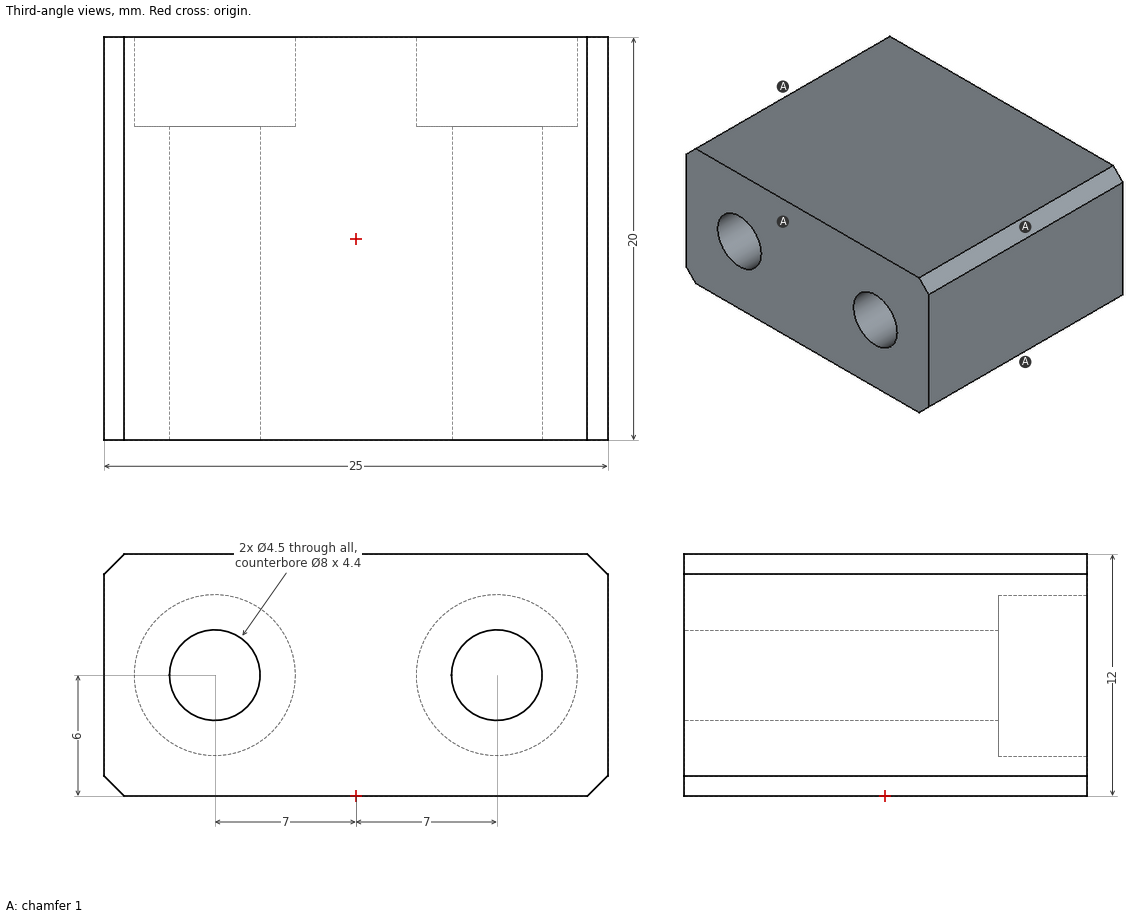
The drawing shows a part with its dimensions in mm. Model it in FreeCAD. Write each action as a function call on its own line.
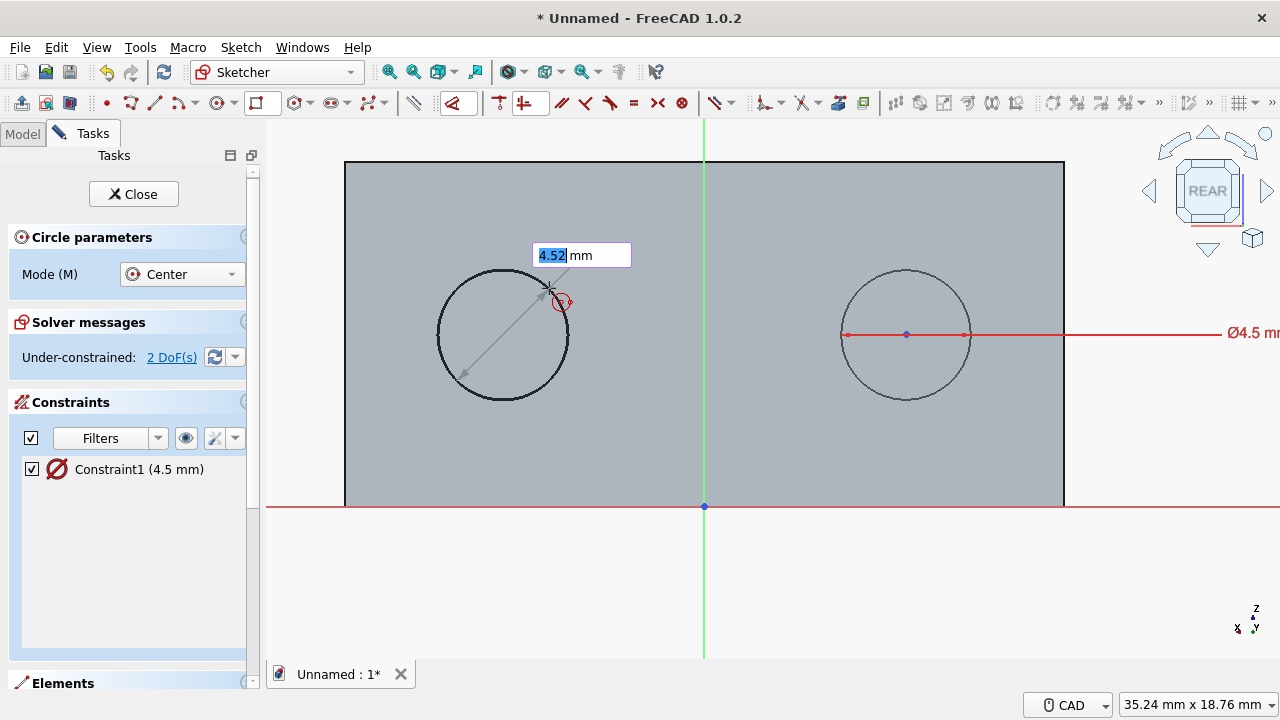
text(4.5)
key(Return)
key(Escape)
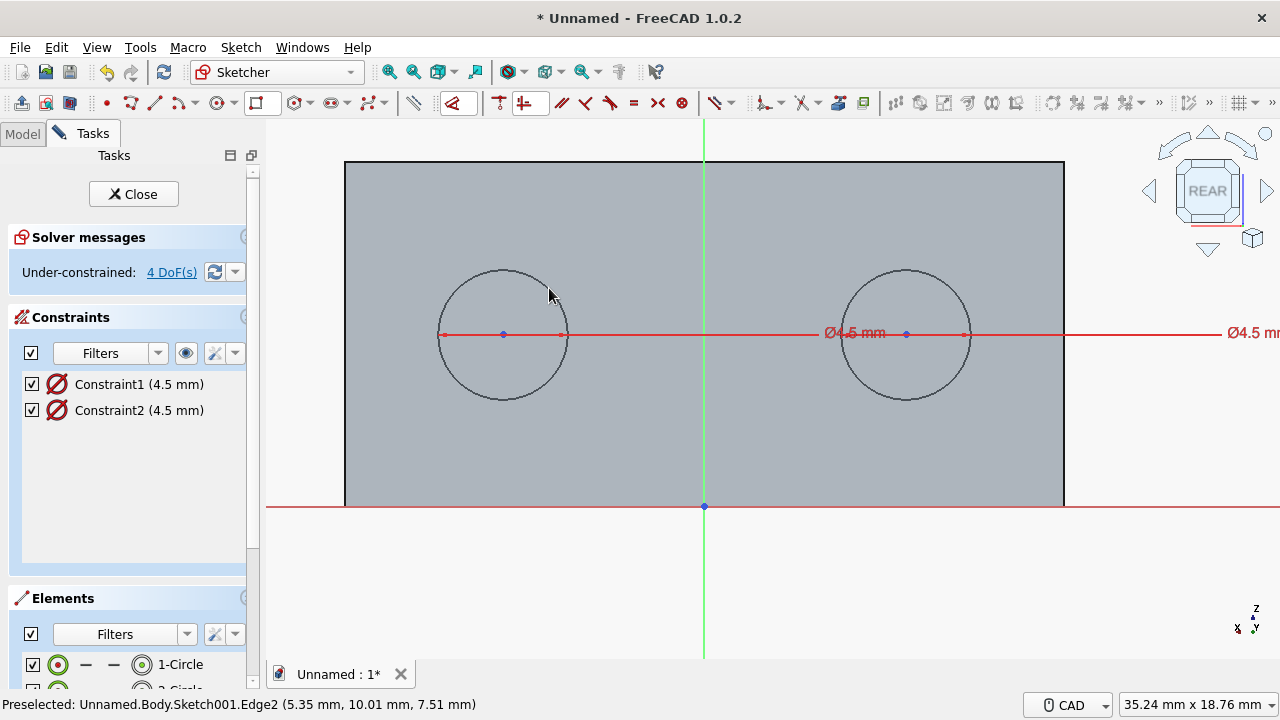
click(906, 335)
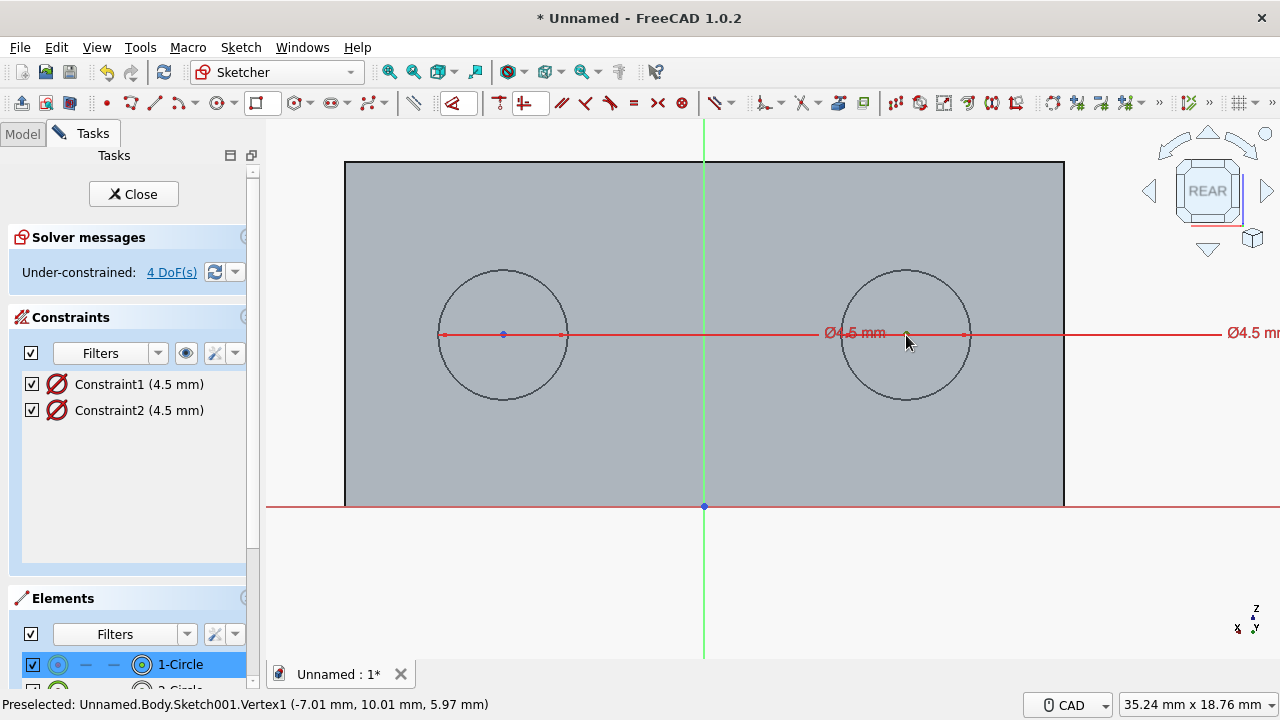
click(503, 335)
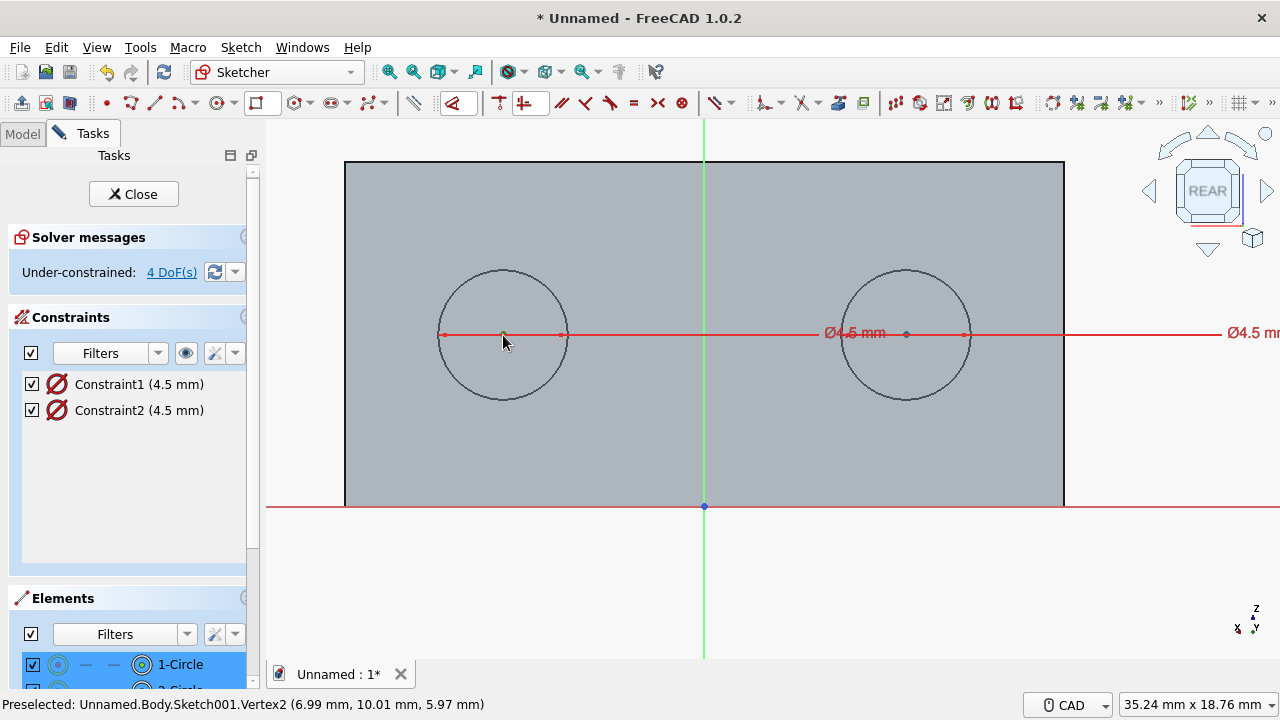
key(h)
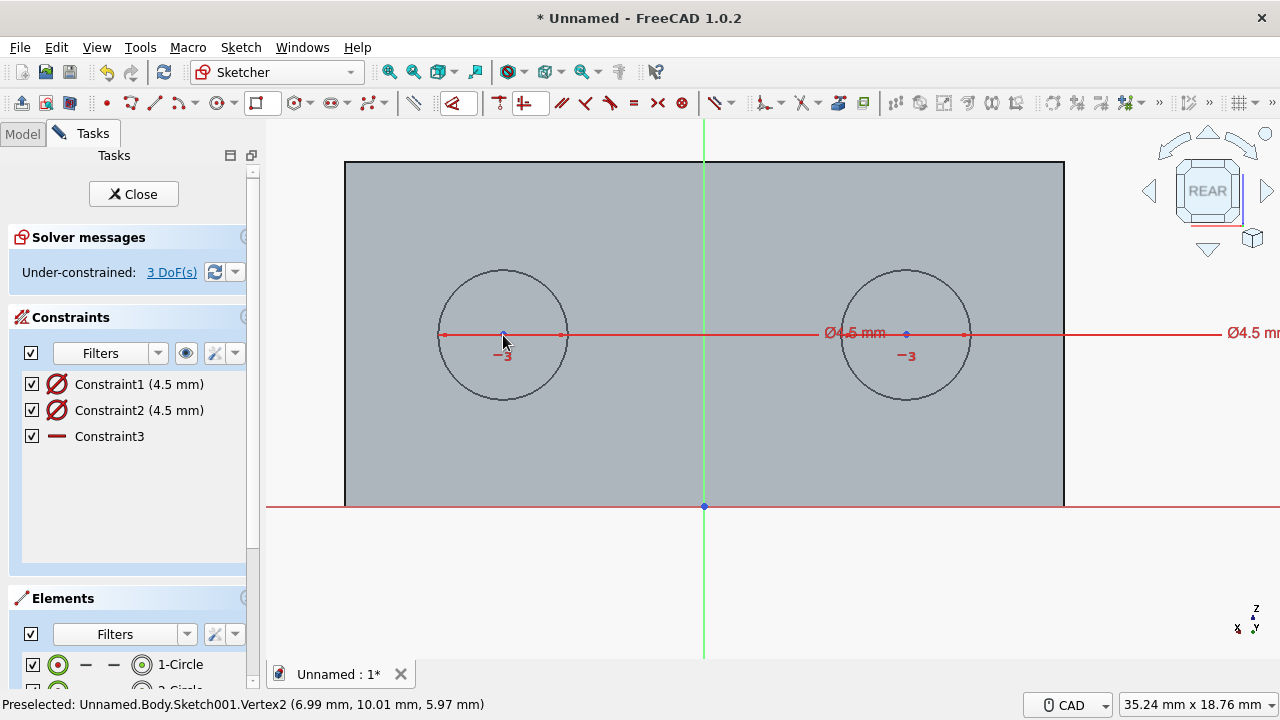
key(d)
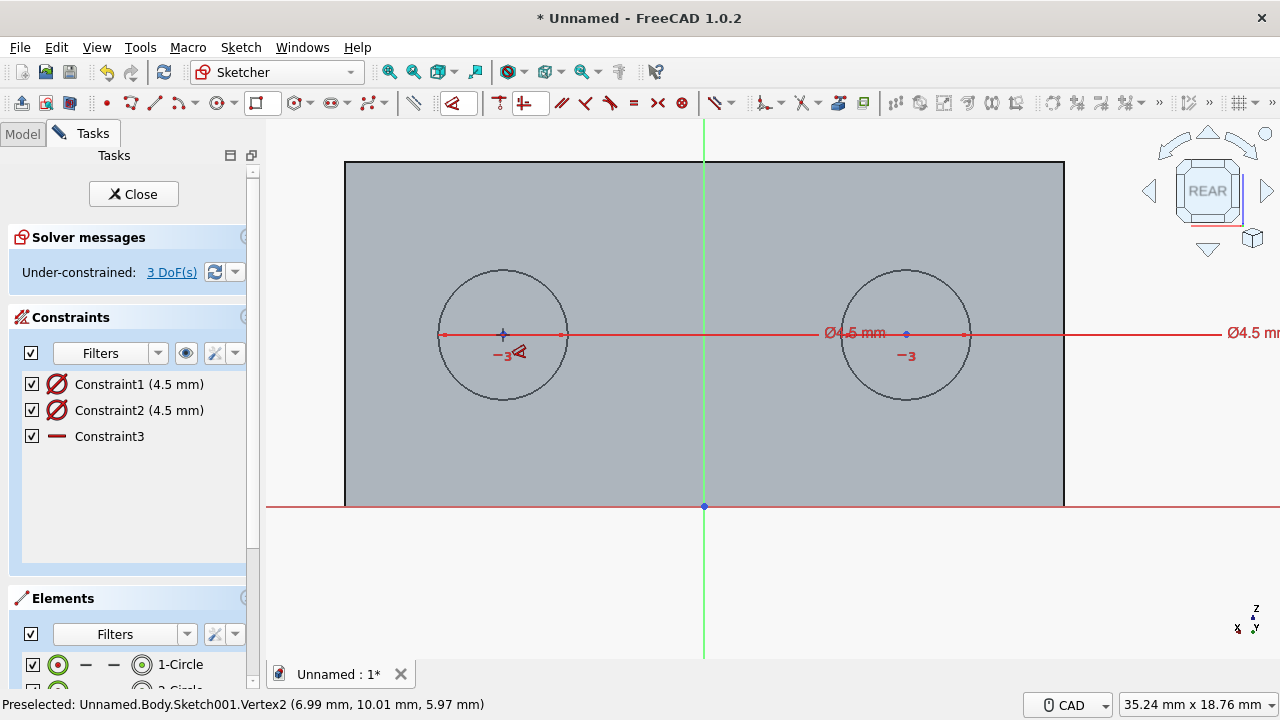
click(906, 335)
click(805, 541)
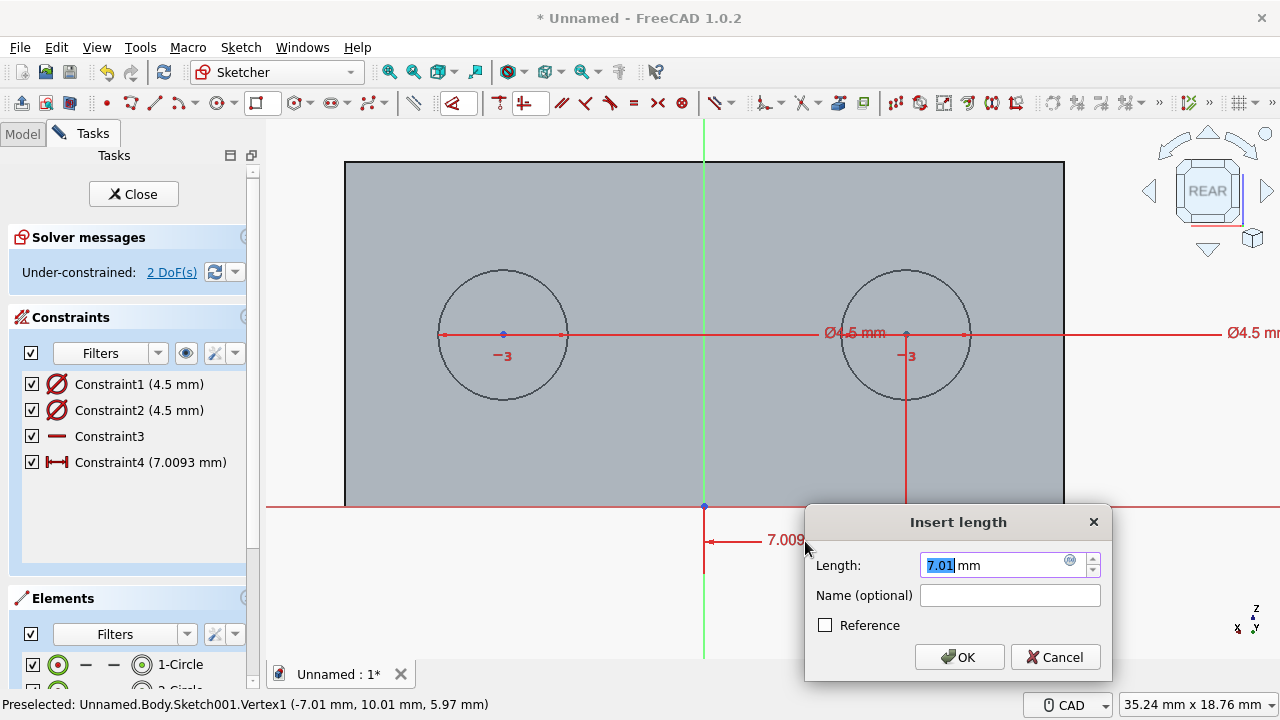
text(7)
key(Return)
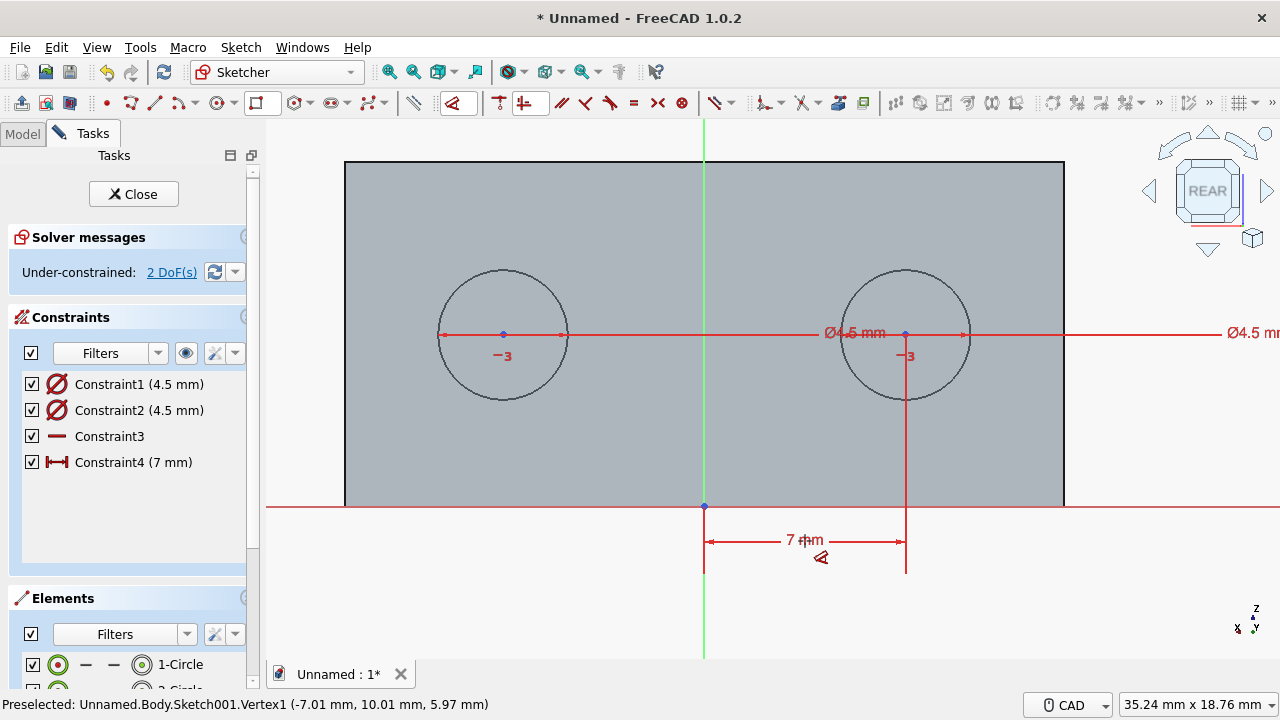
click(906, 335)
click(940, 421)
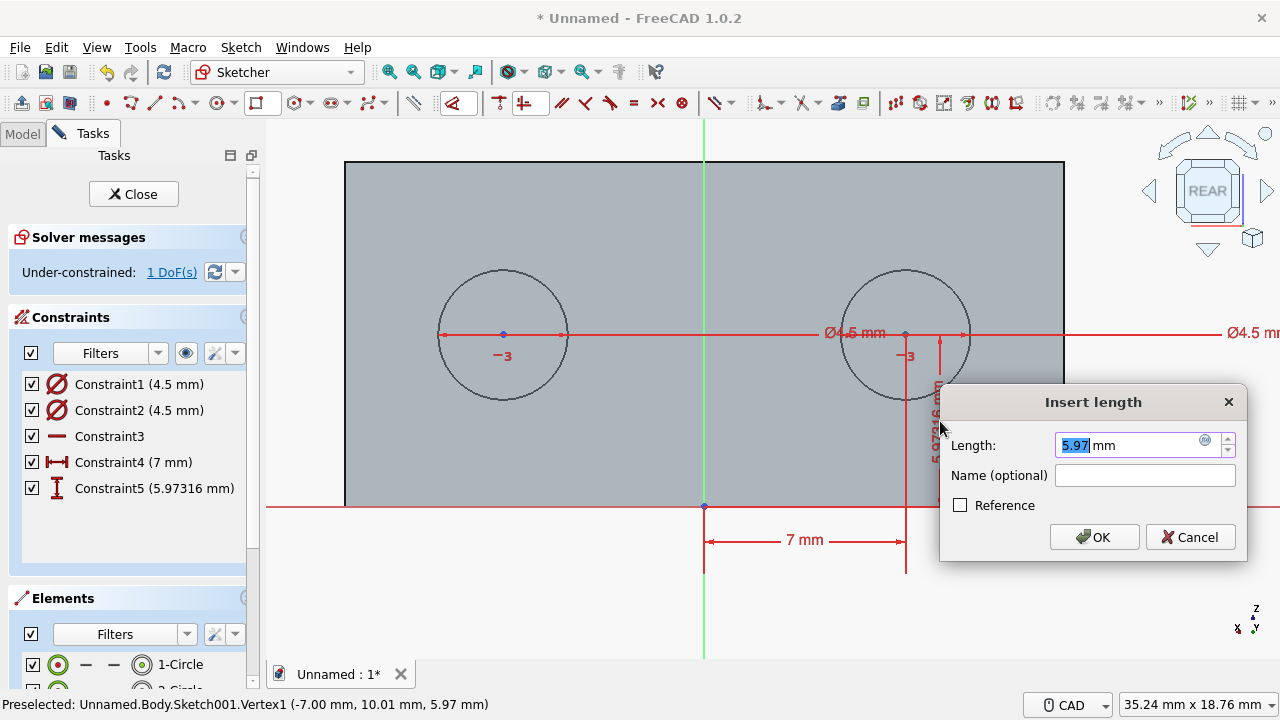
text(6)
key(Return)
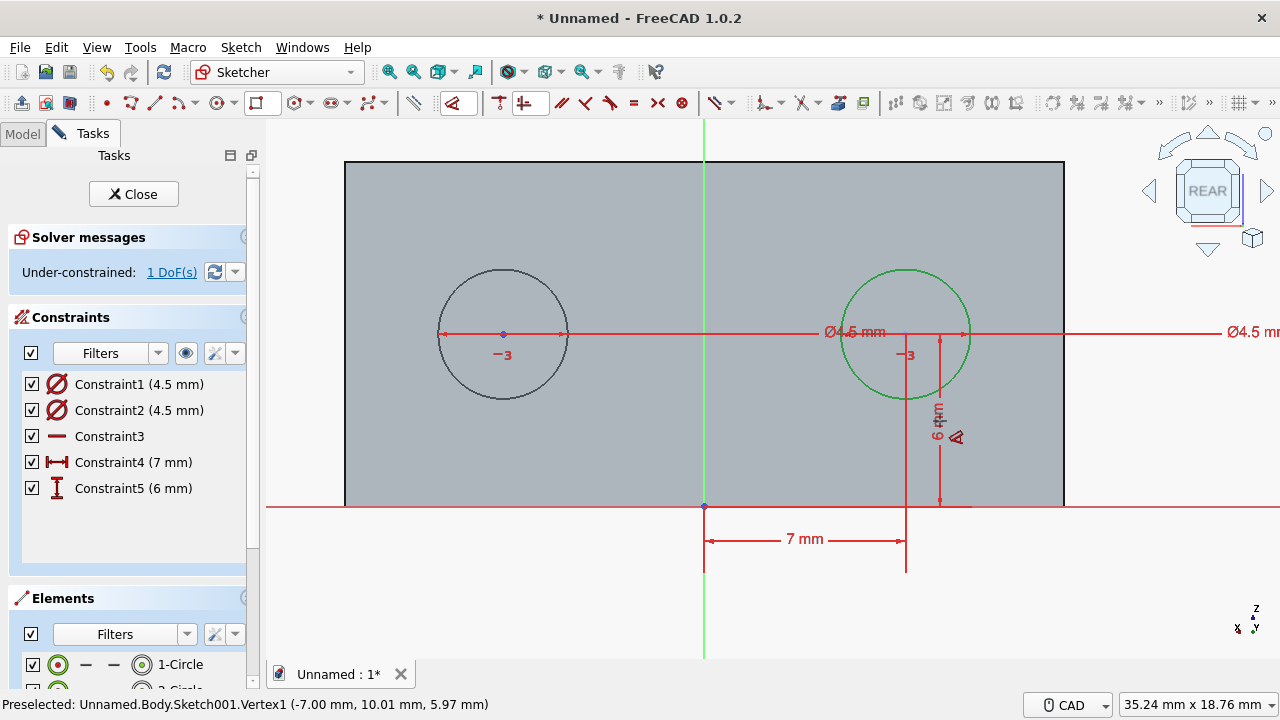
click(503, 334)
click(604, 541)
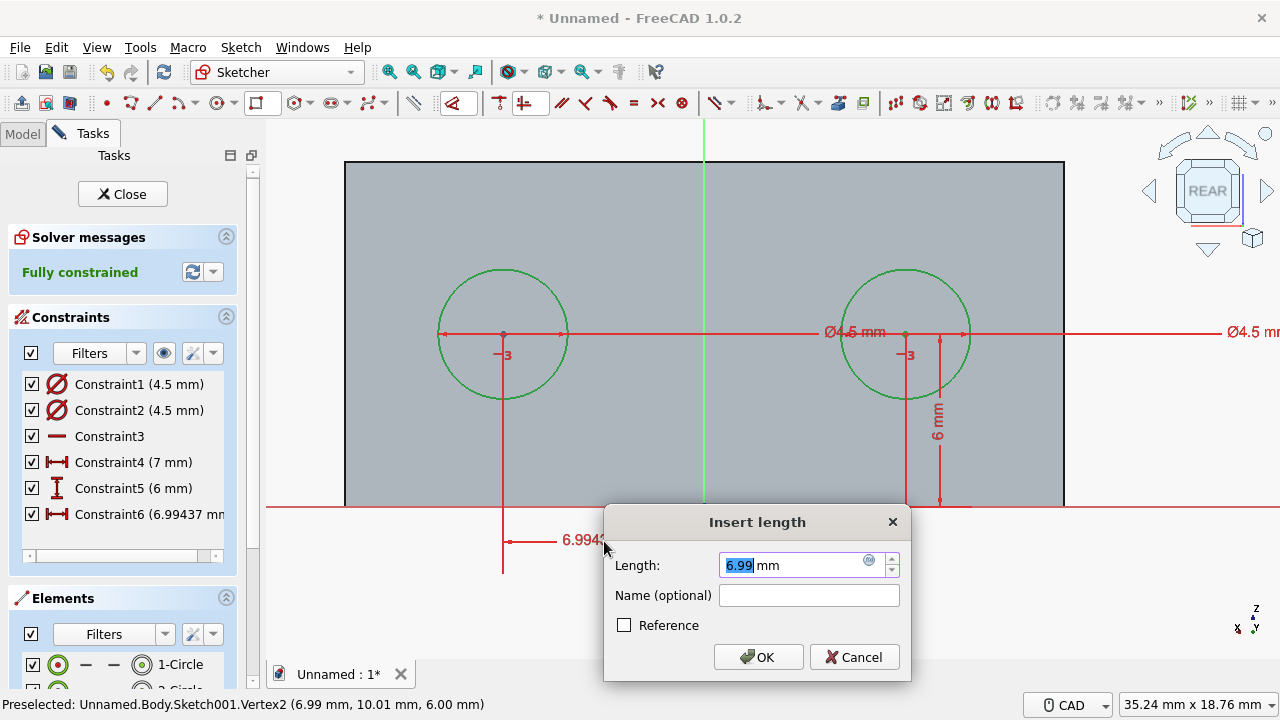
text(7)
key(Return)
key(Escape)